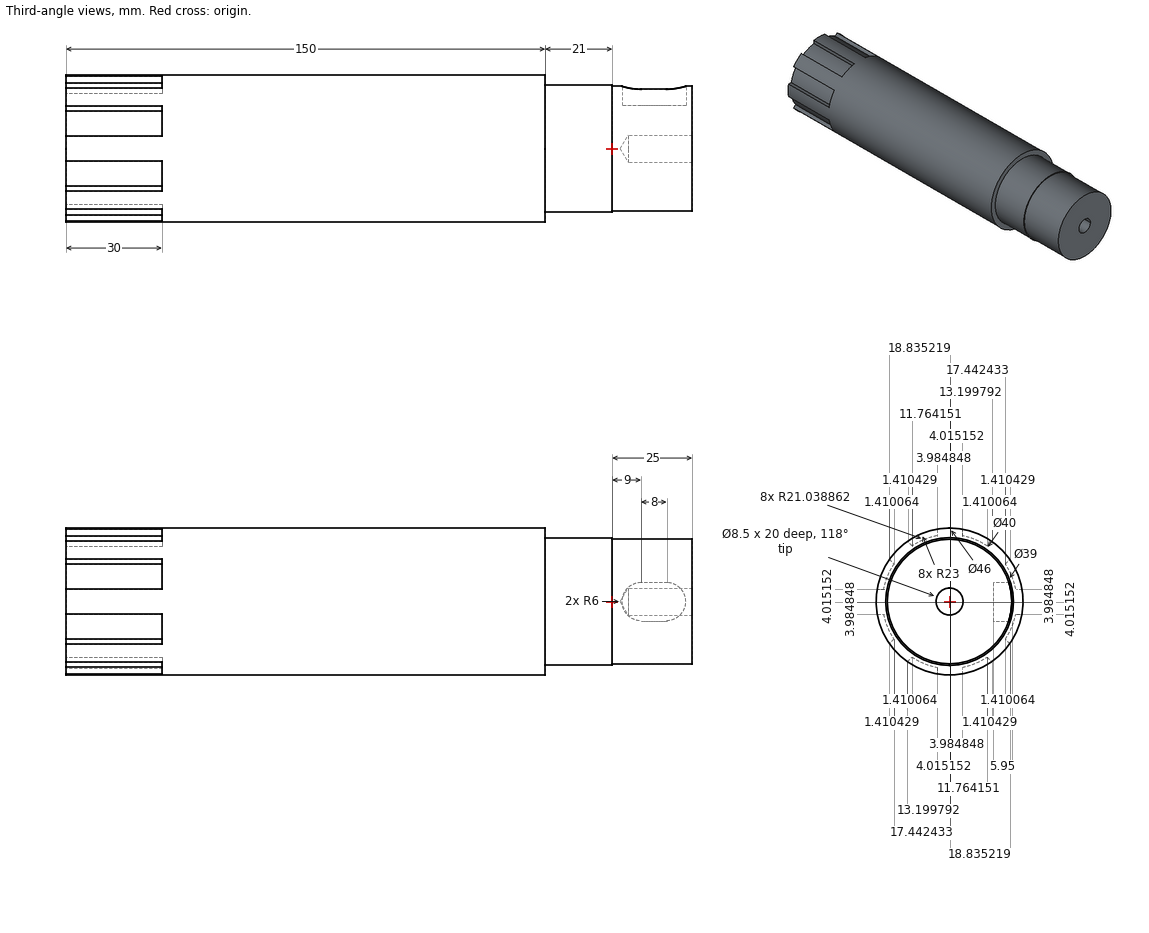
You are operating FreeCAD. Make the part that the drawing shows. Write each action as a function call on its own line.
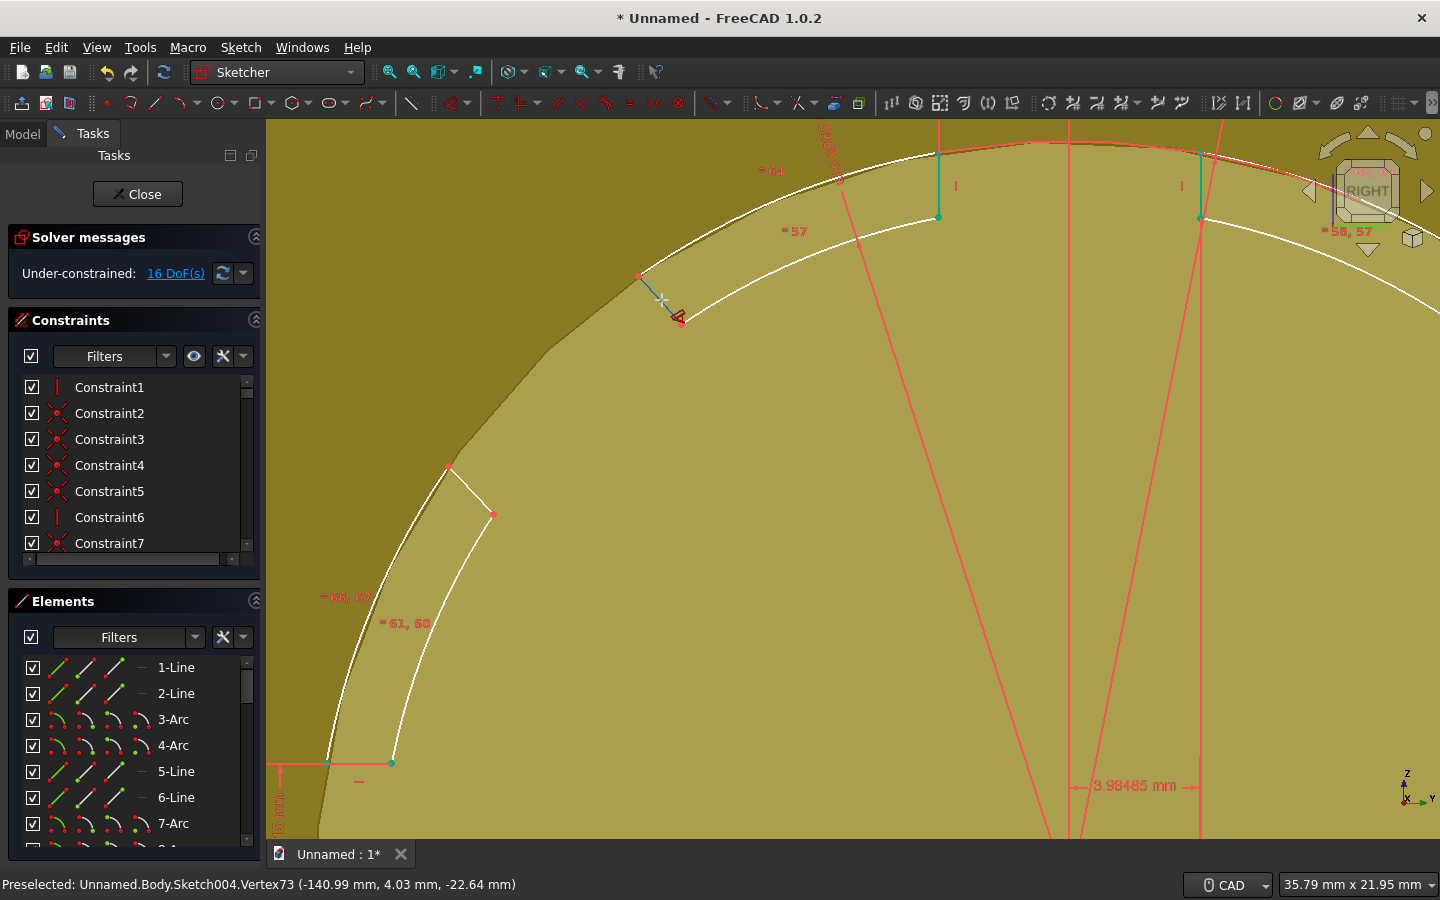
click(660, 300)
click(660, 242)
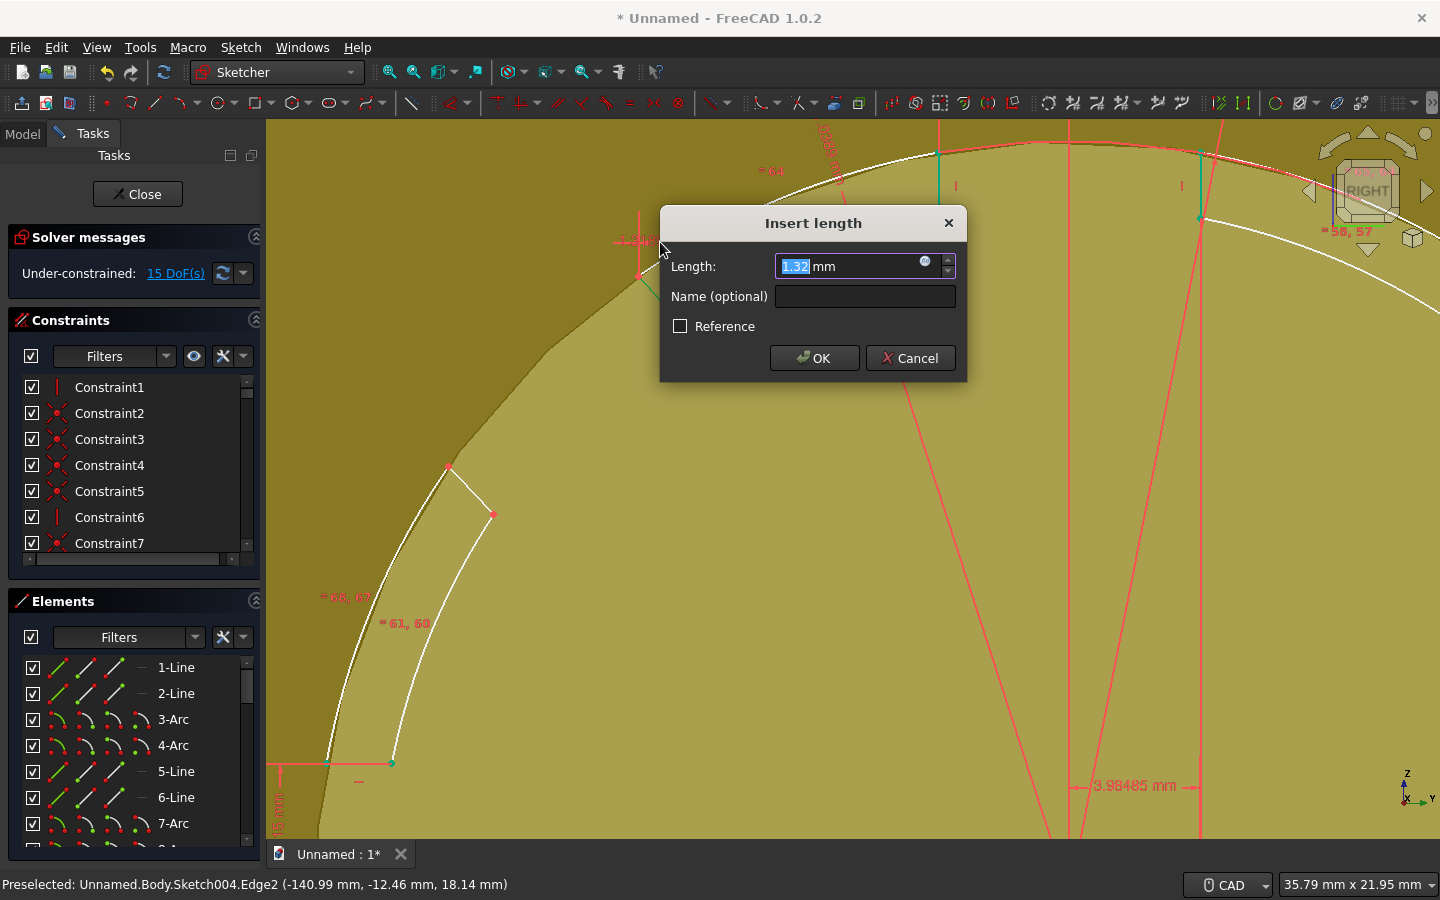
text(1.410429)
key(Return)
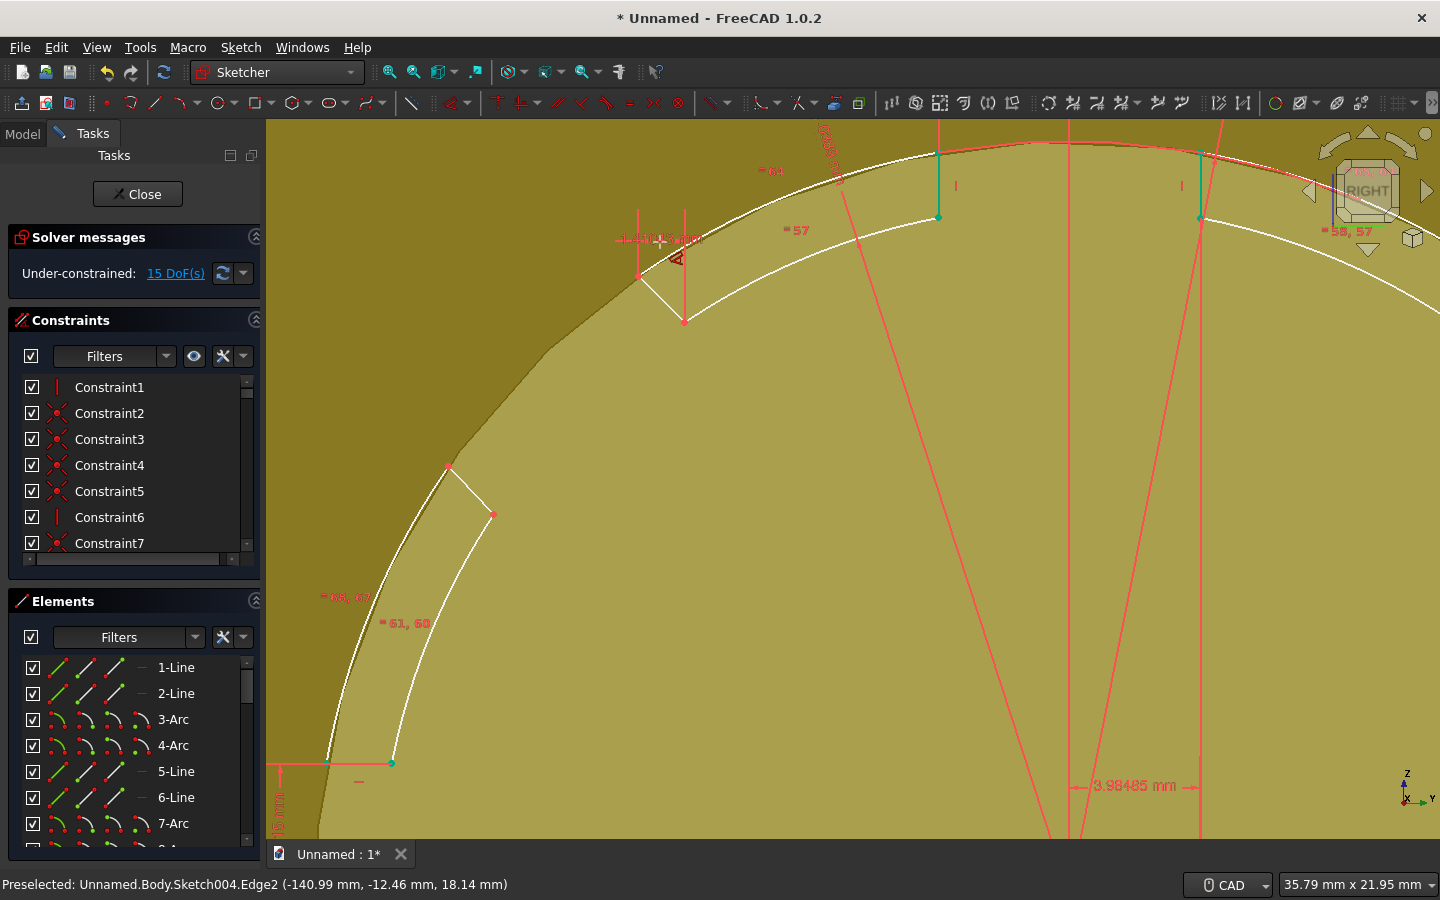
scroll(662, 299, down, 6)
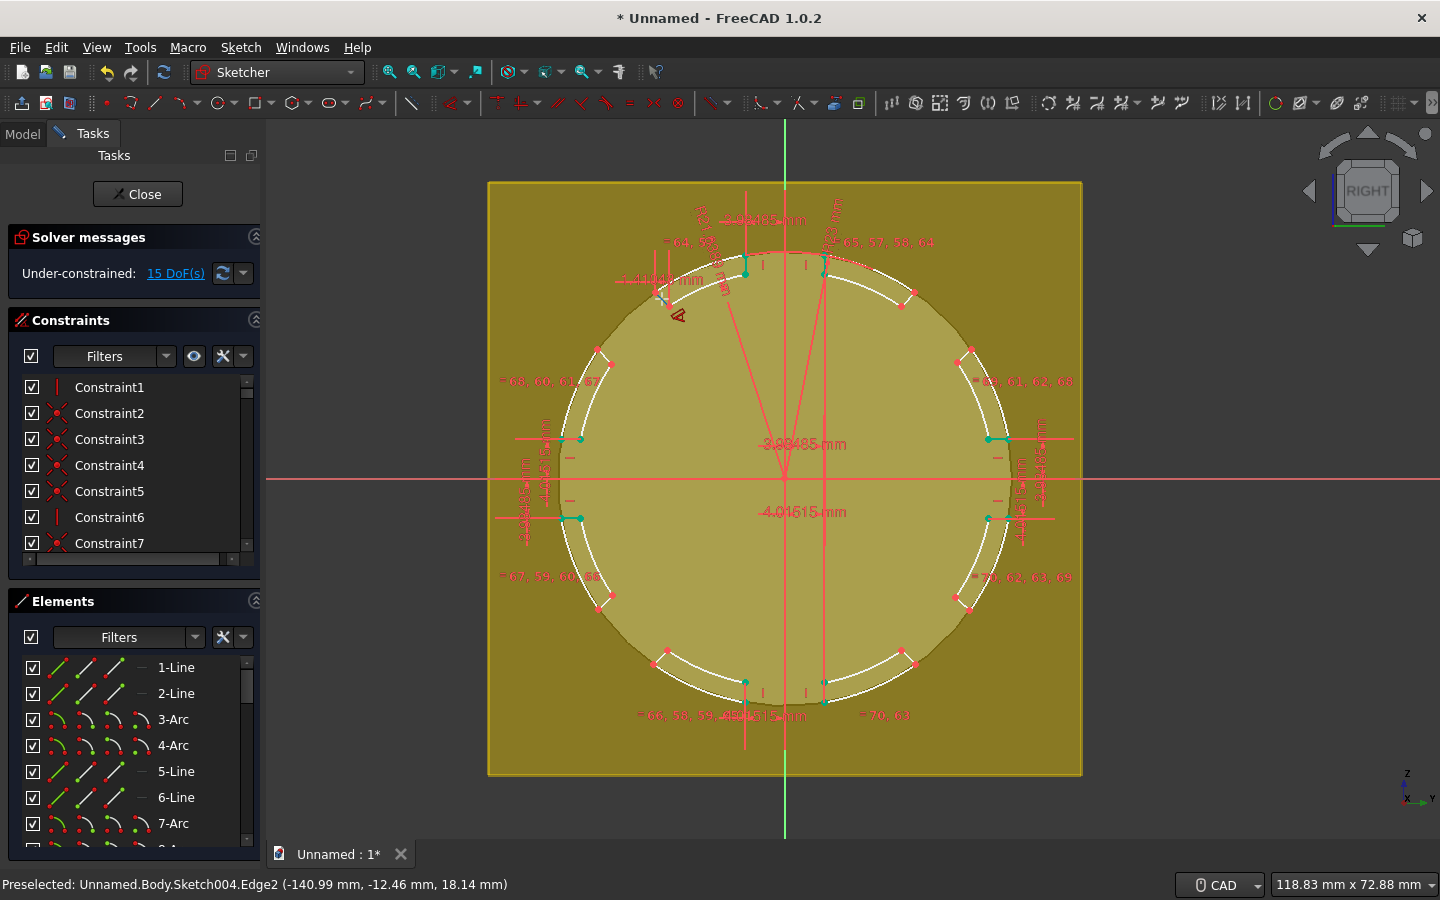
scroll(911, 297, up, 6)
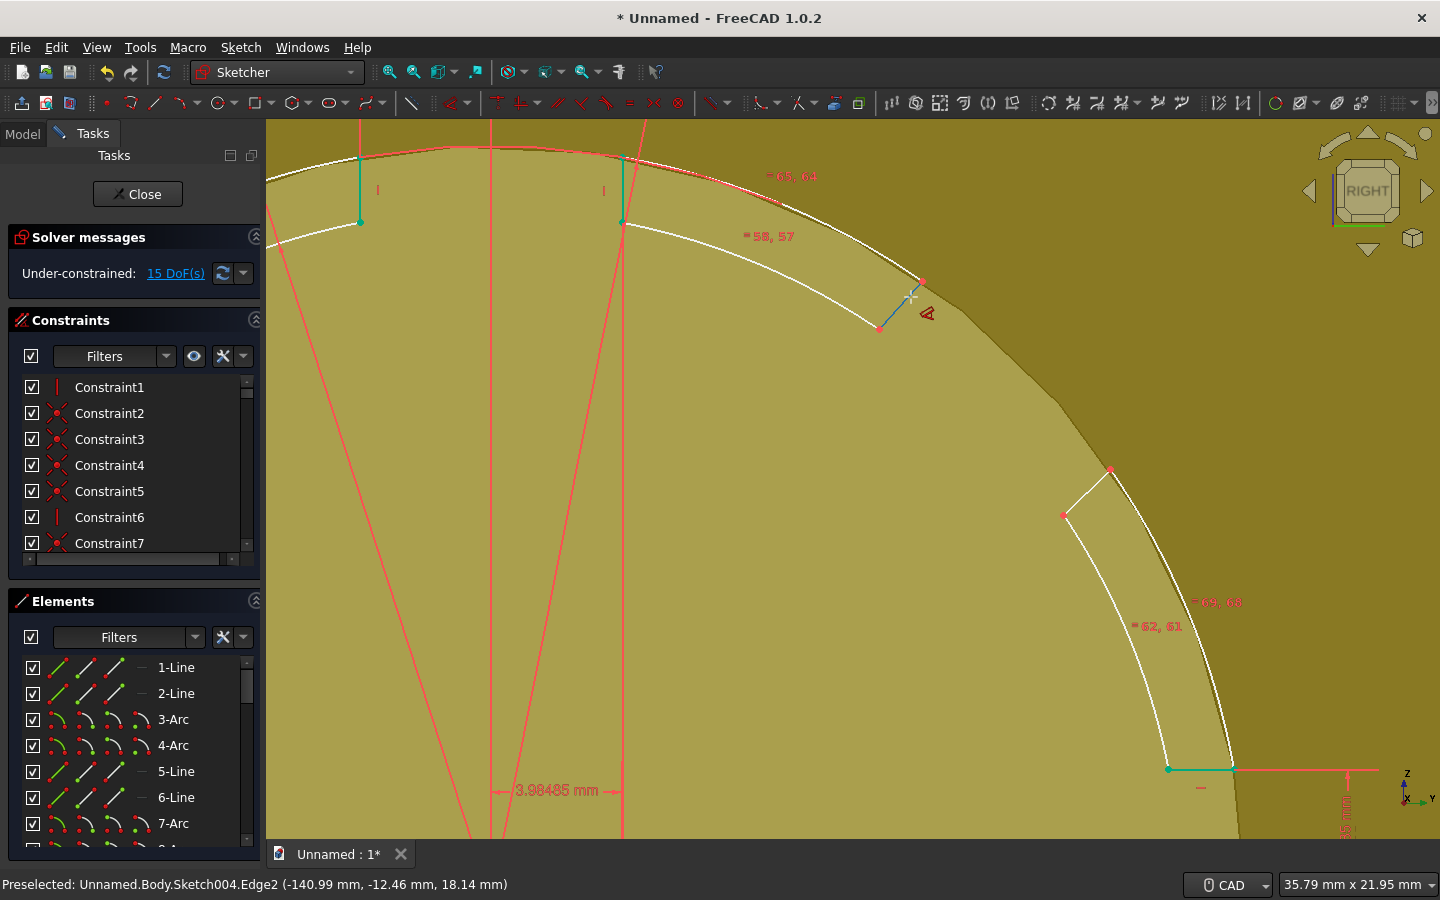
click(909, 296)
click(901, 247)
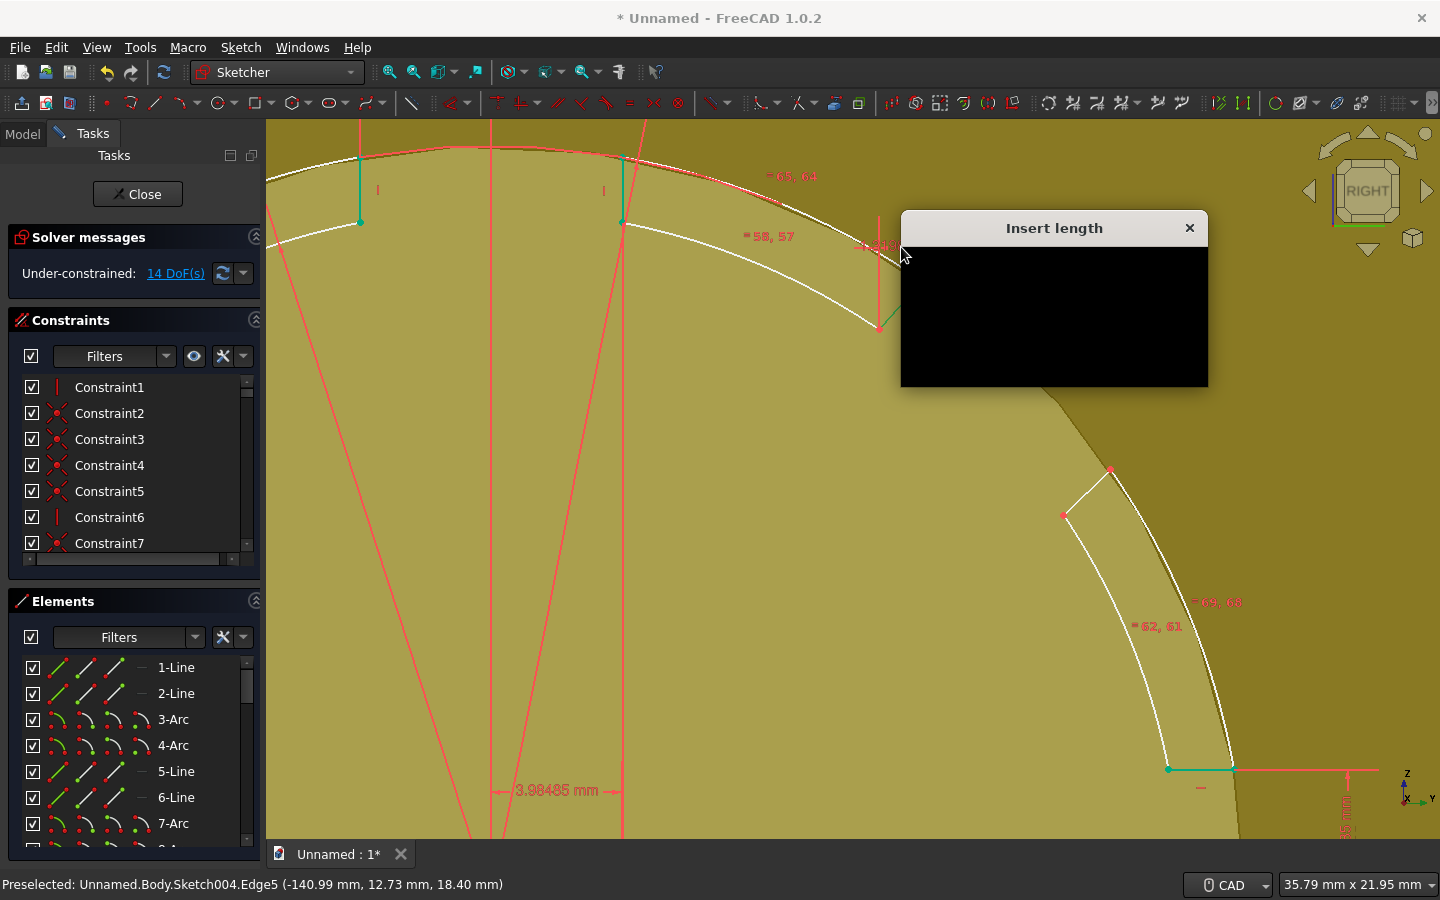
text(1.410064)
key(Return)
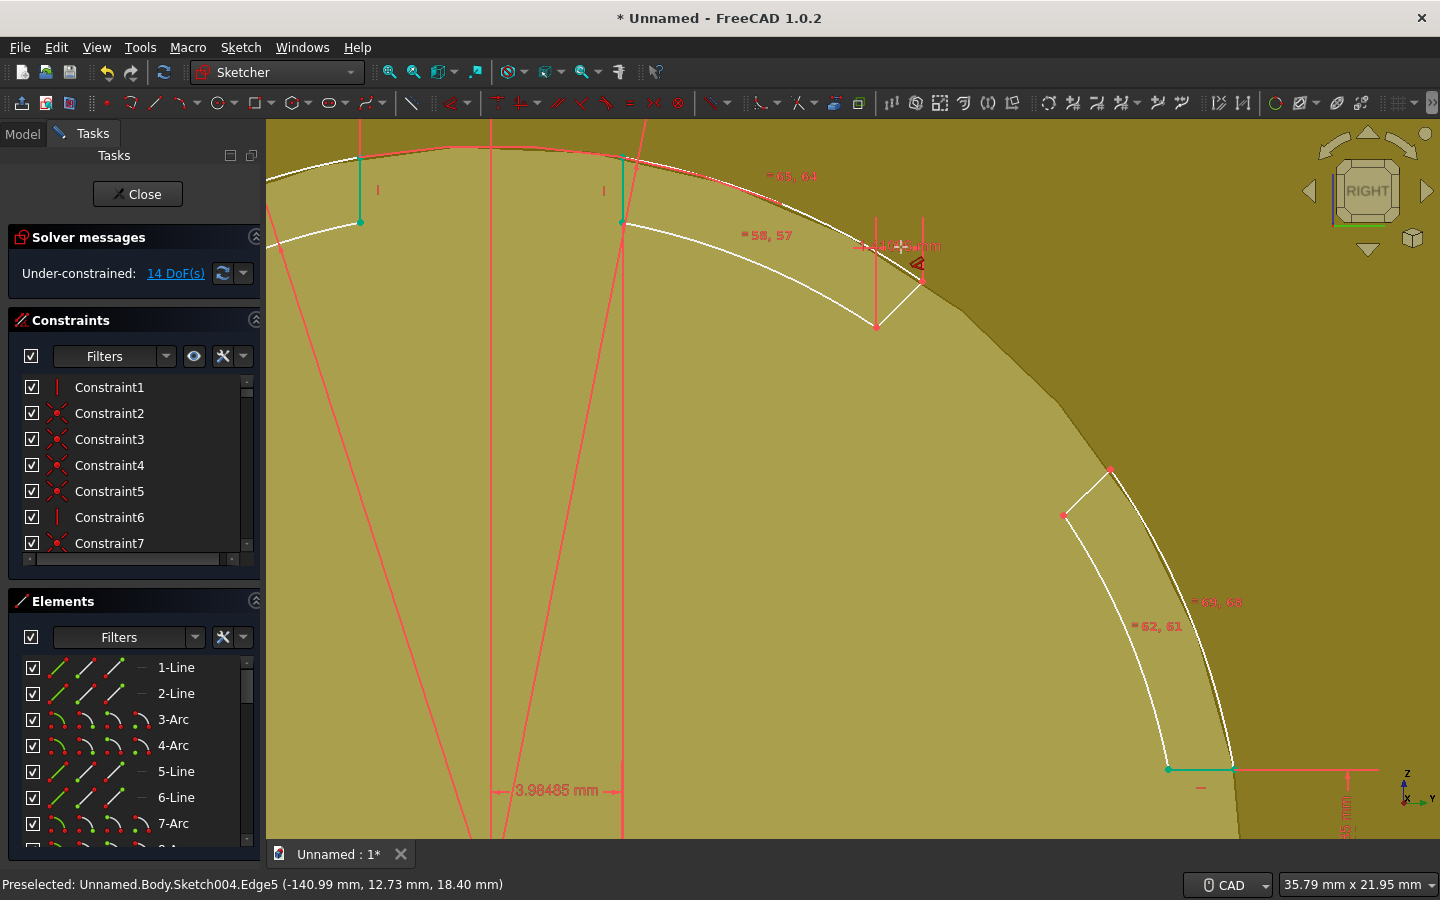
scroll(911, 297, down, 6)